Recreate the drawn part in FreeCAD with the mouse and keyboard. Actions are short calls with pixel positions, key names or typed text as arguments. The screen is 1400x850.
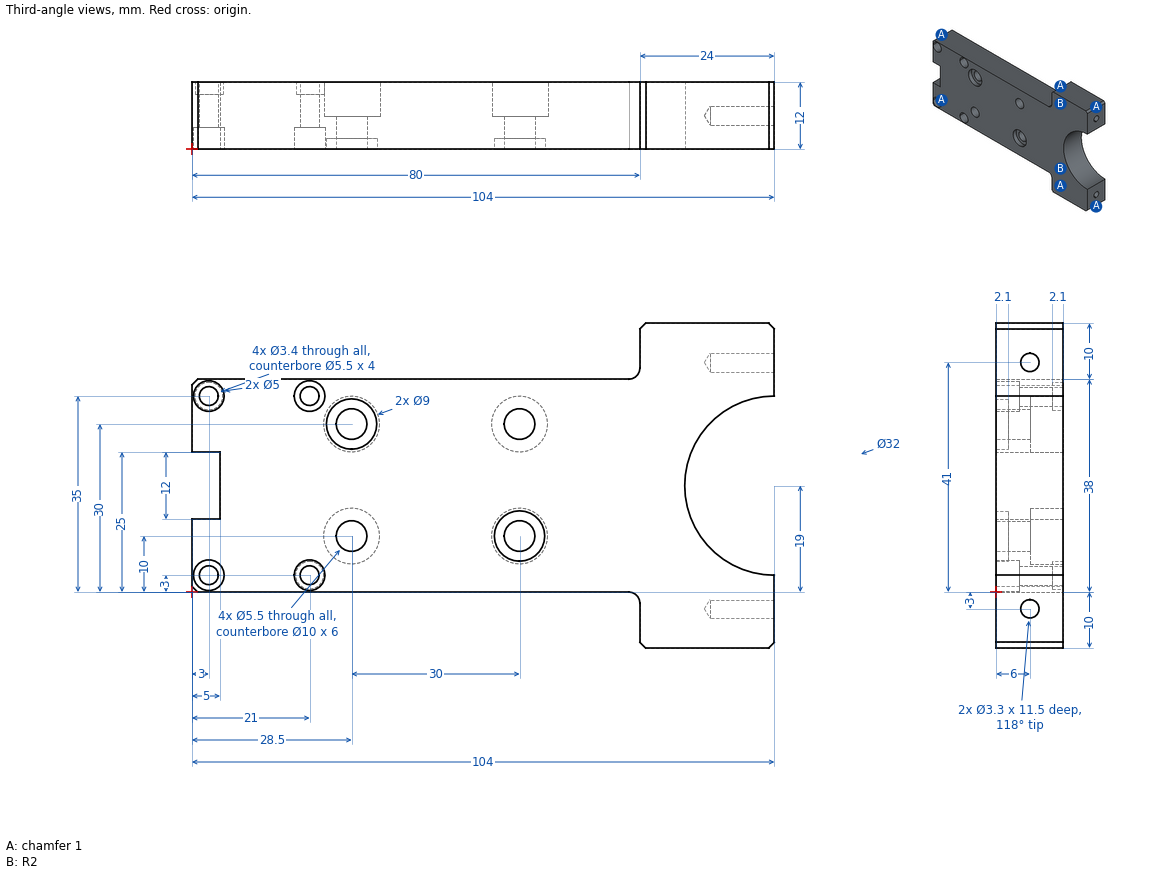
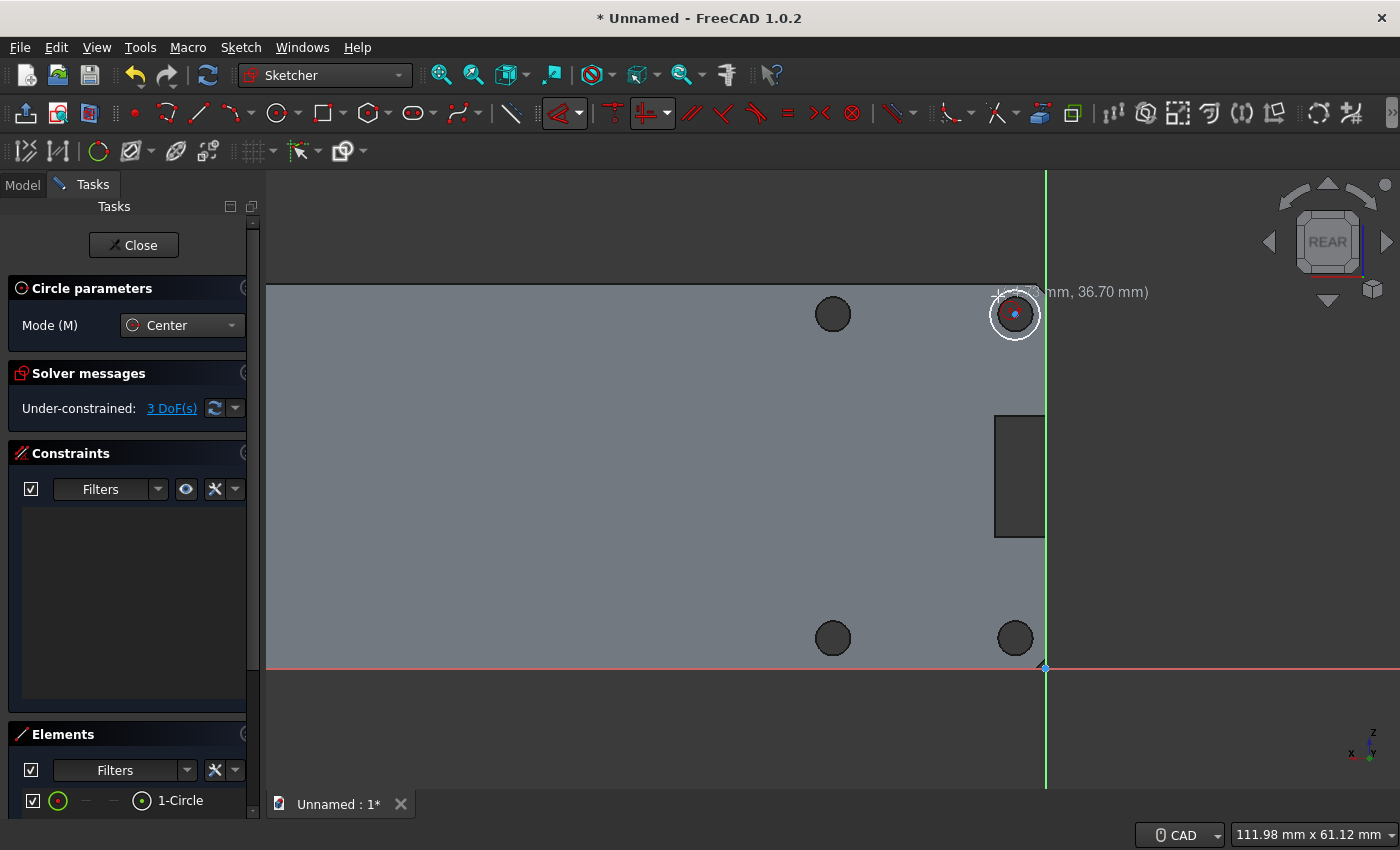
click(833, 638)
click(851, 620)
key(Escape)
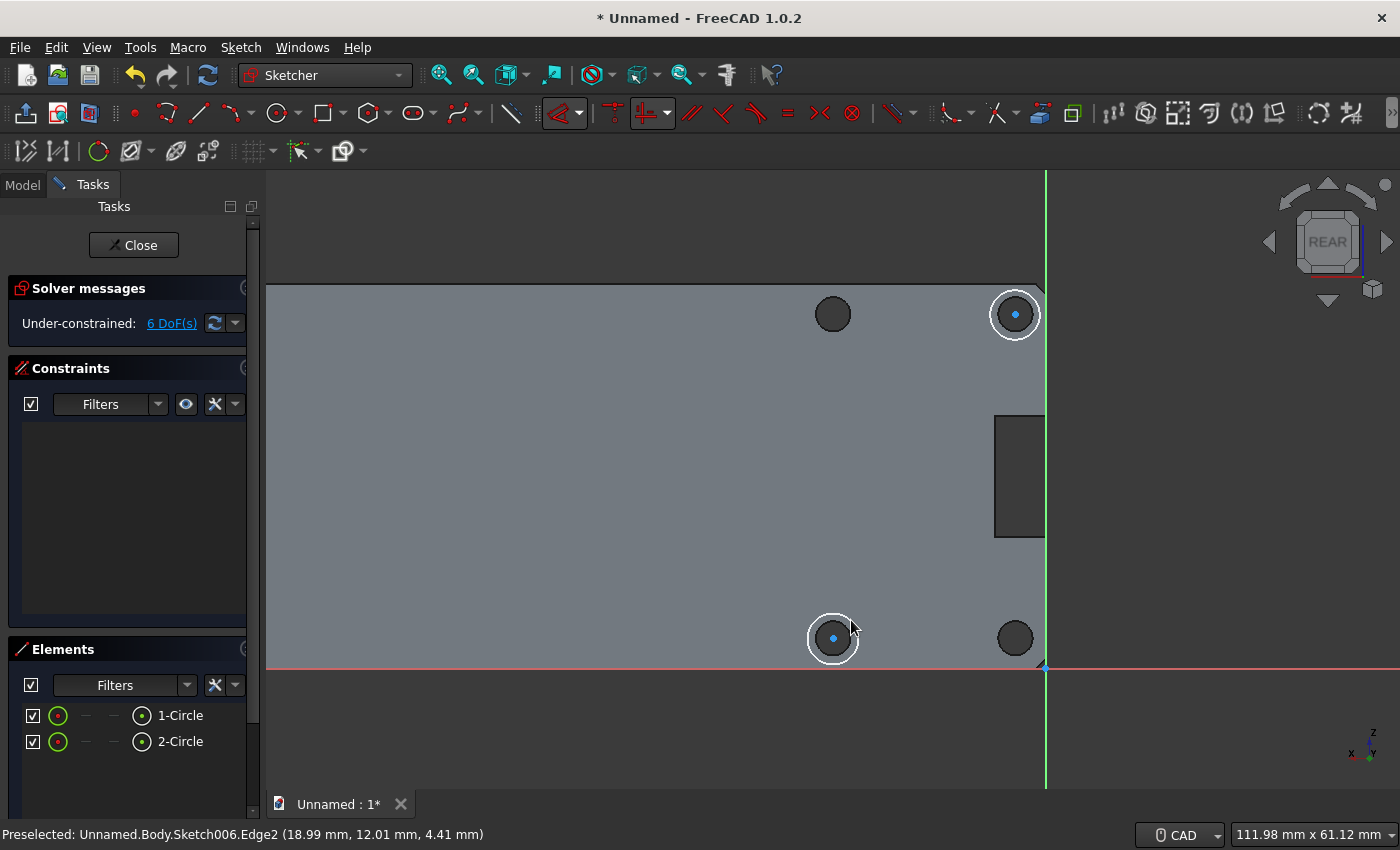
click(1032, 297)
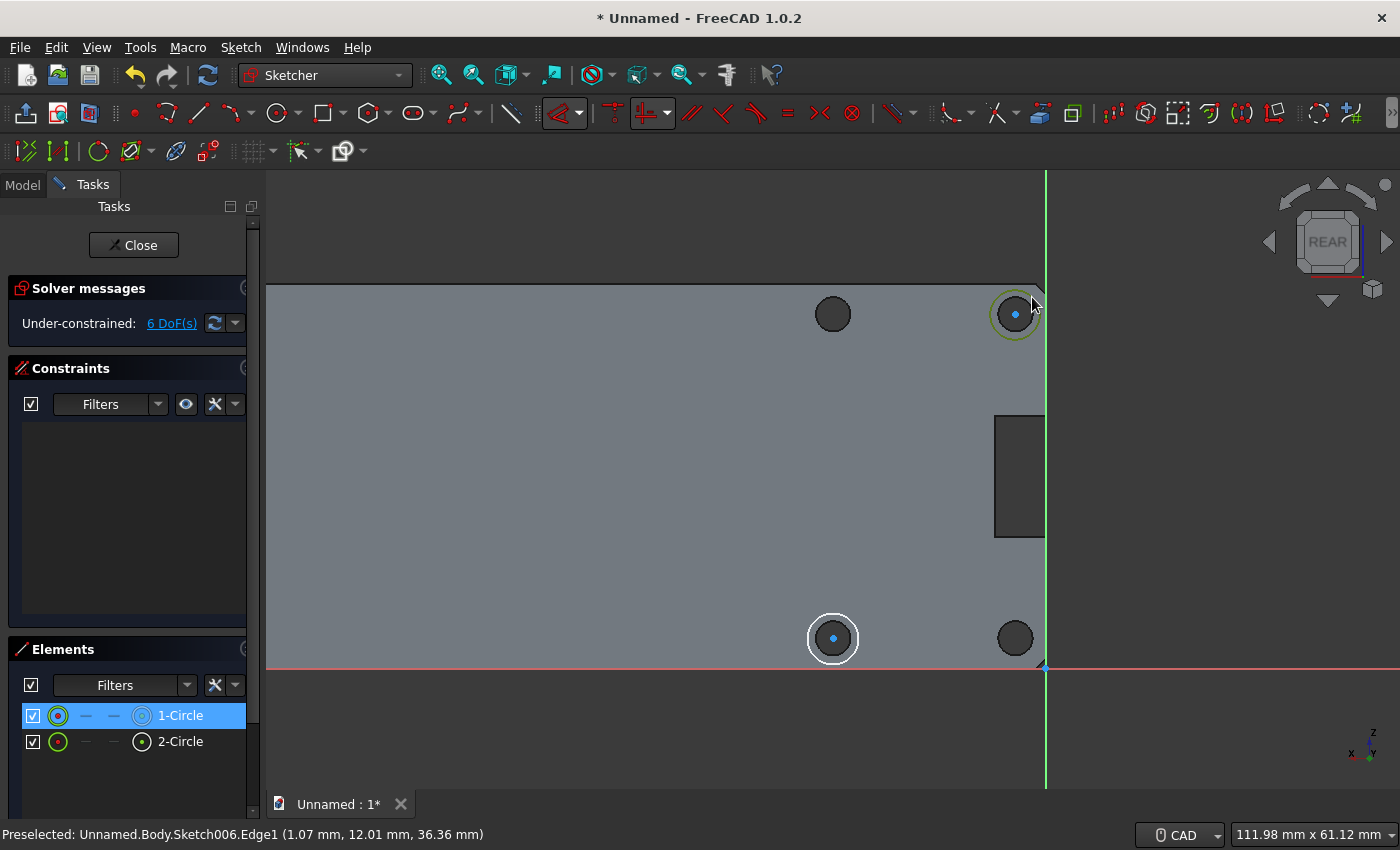
click(851, 621)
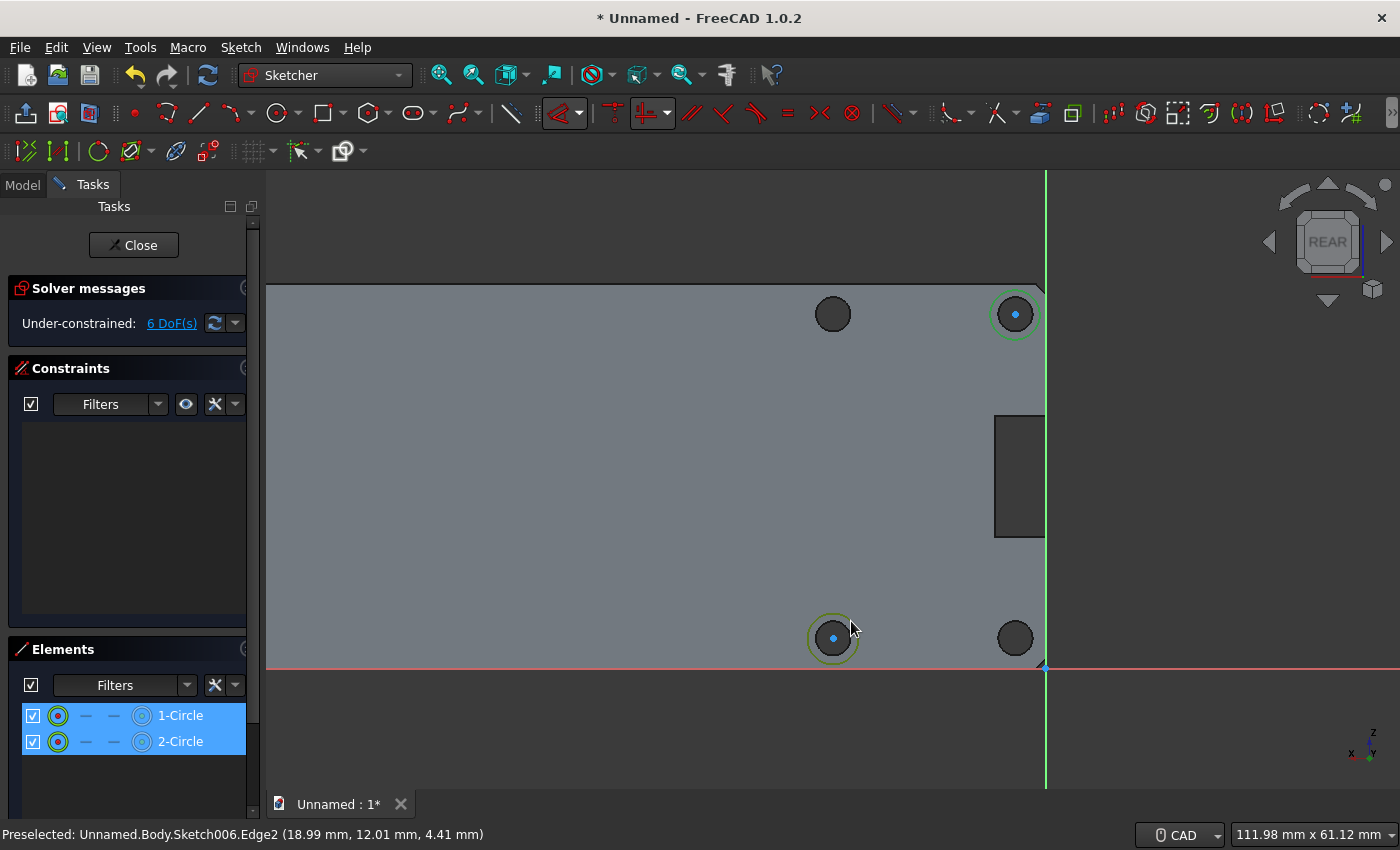
click(788, 114)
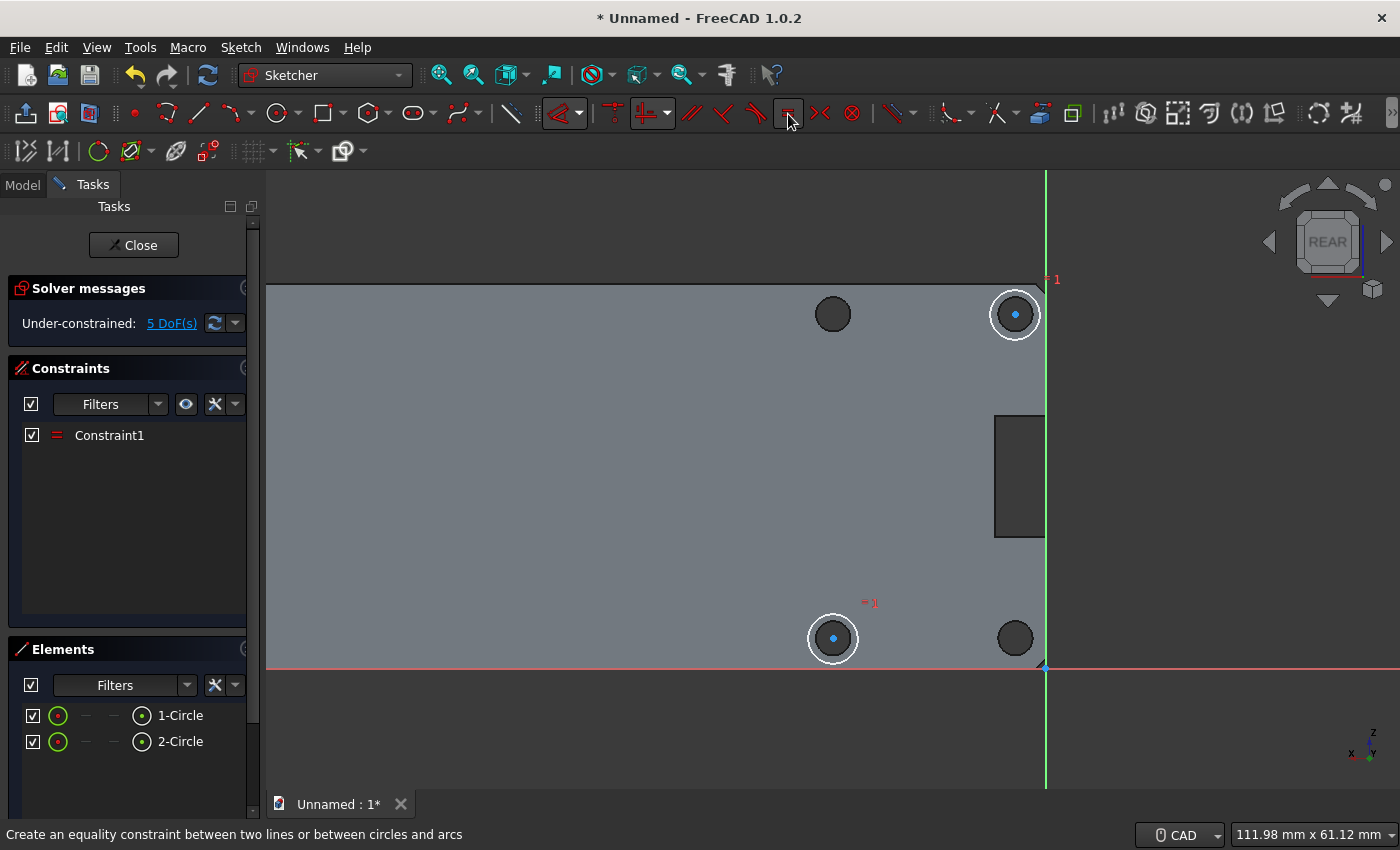
click(1032, 297)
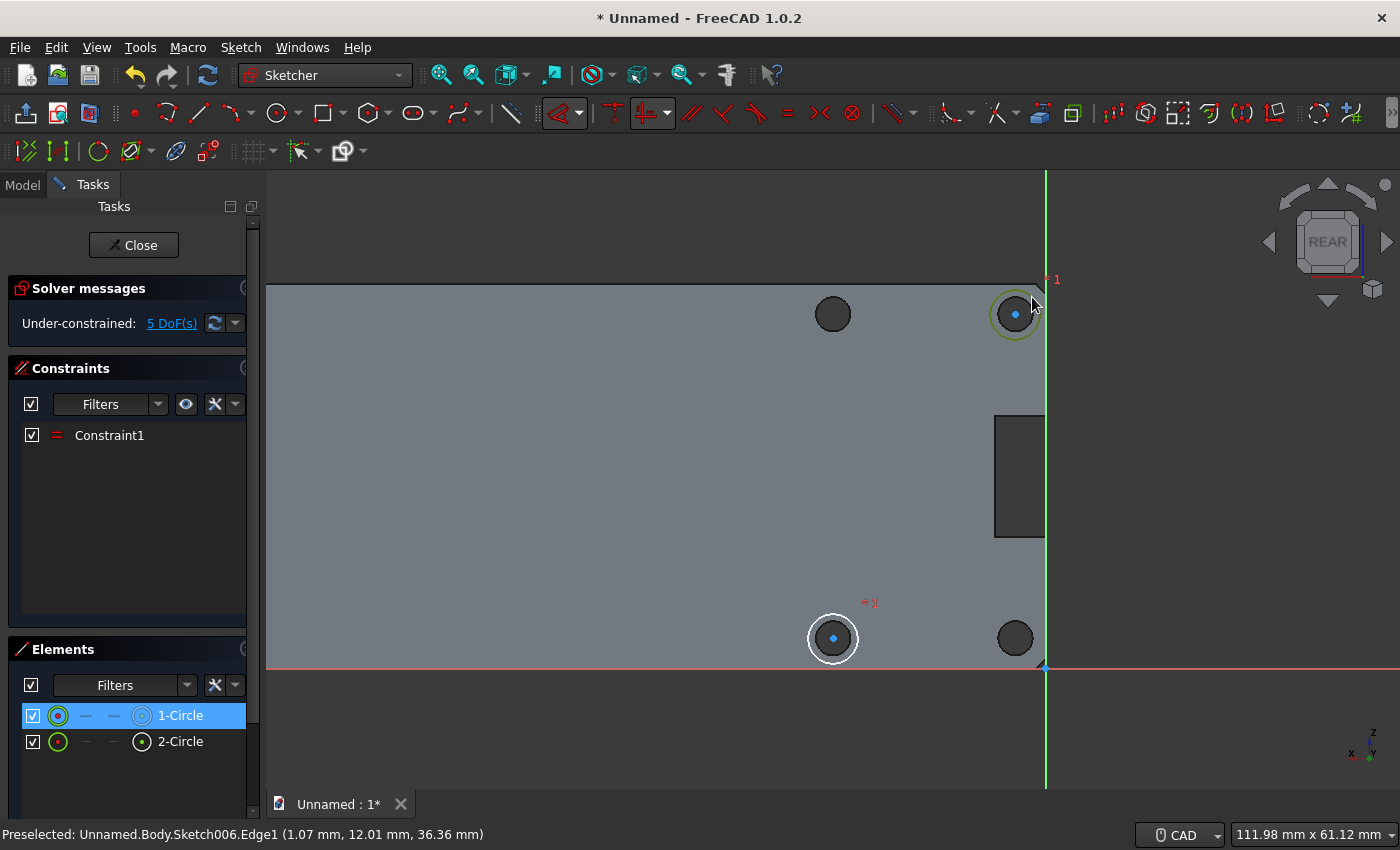
click(582, 114)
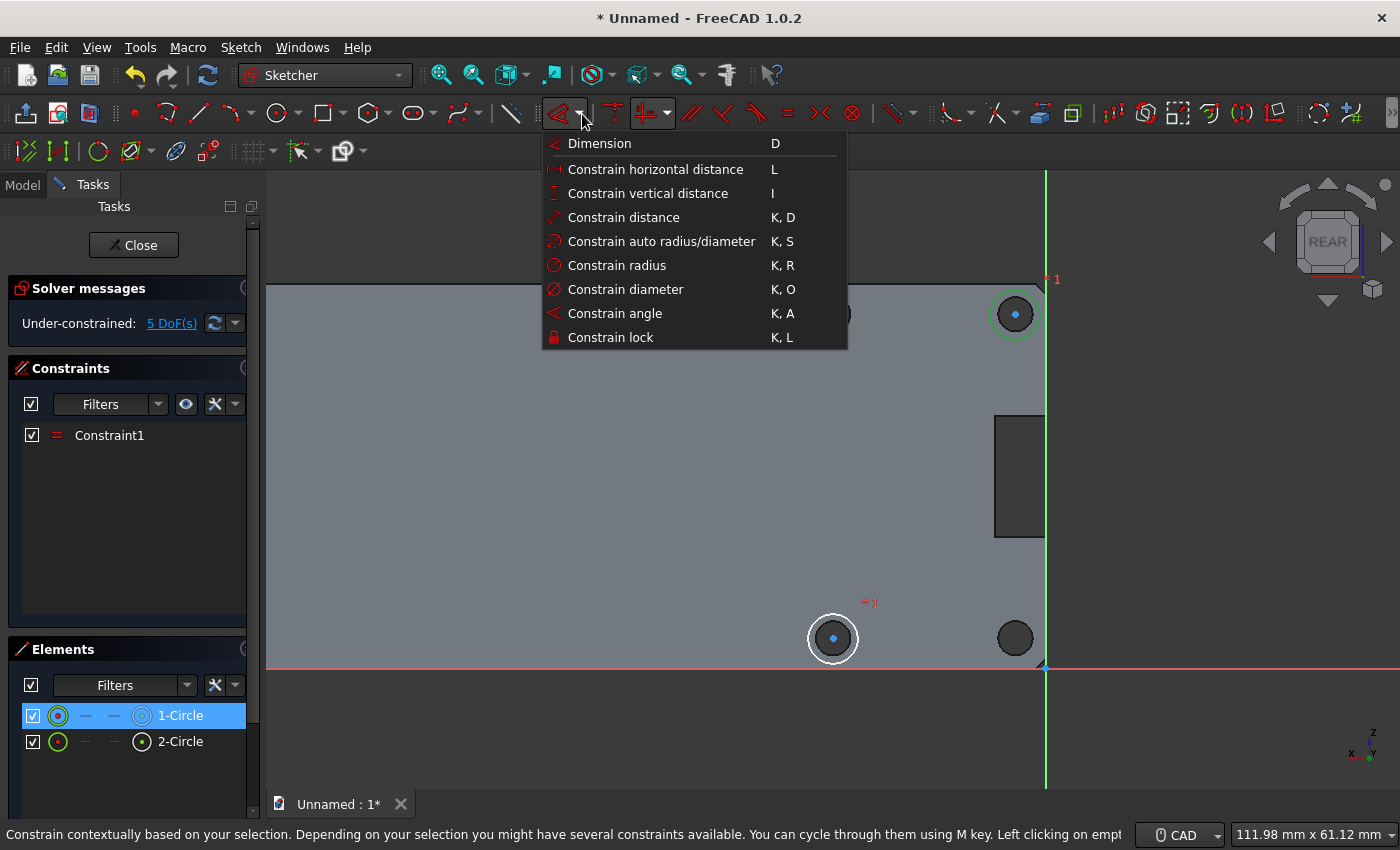
click(695, 289)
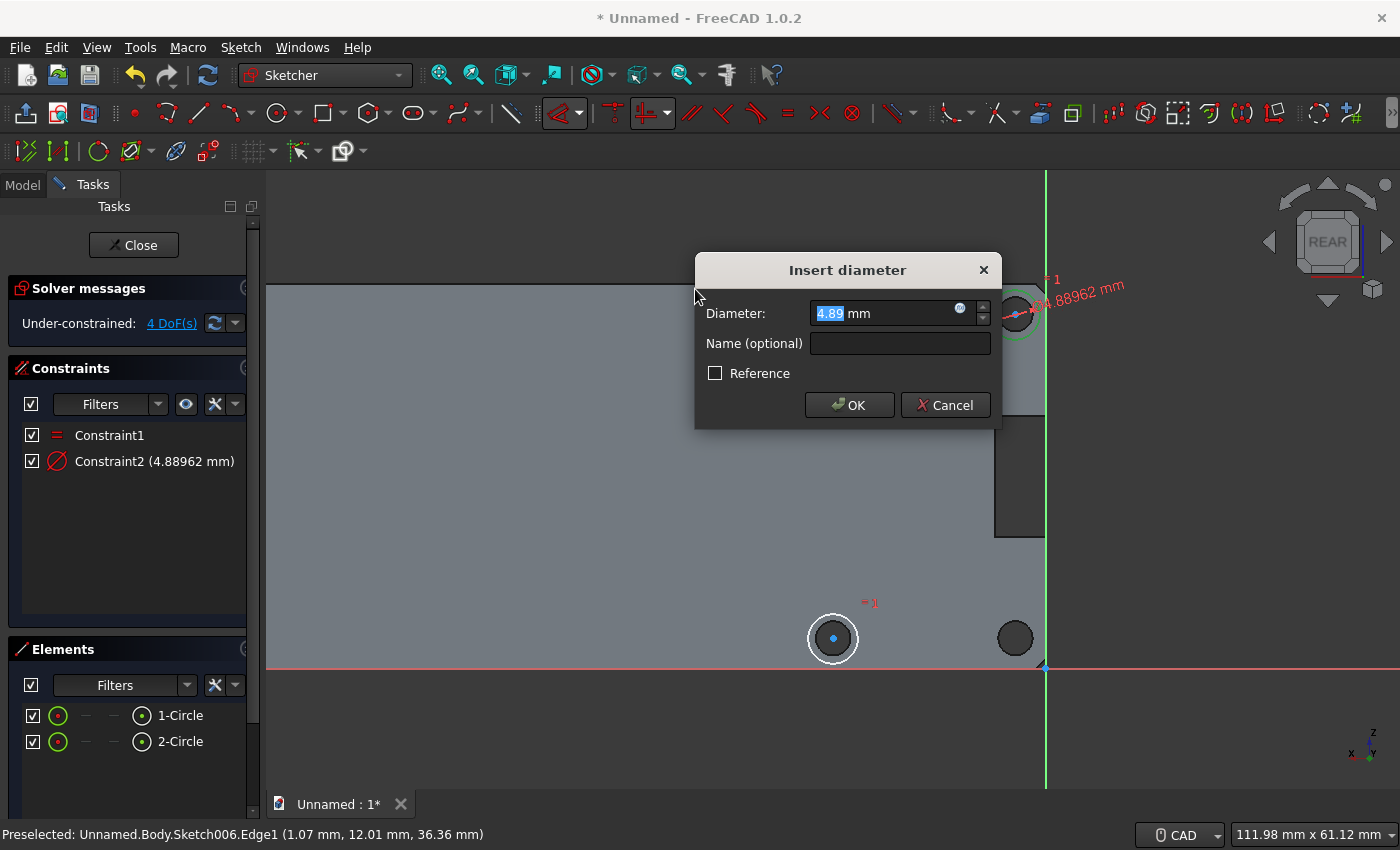
text(5)
key(Return)